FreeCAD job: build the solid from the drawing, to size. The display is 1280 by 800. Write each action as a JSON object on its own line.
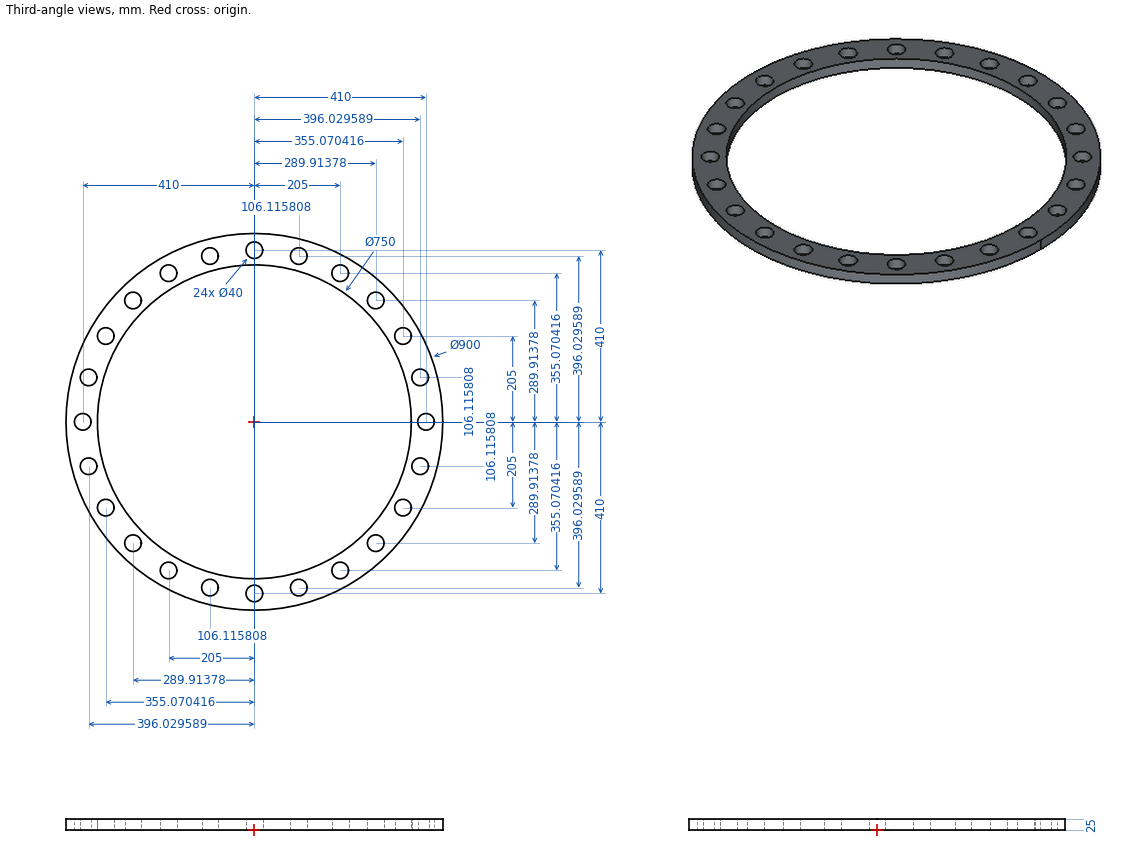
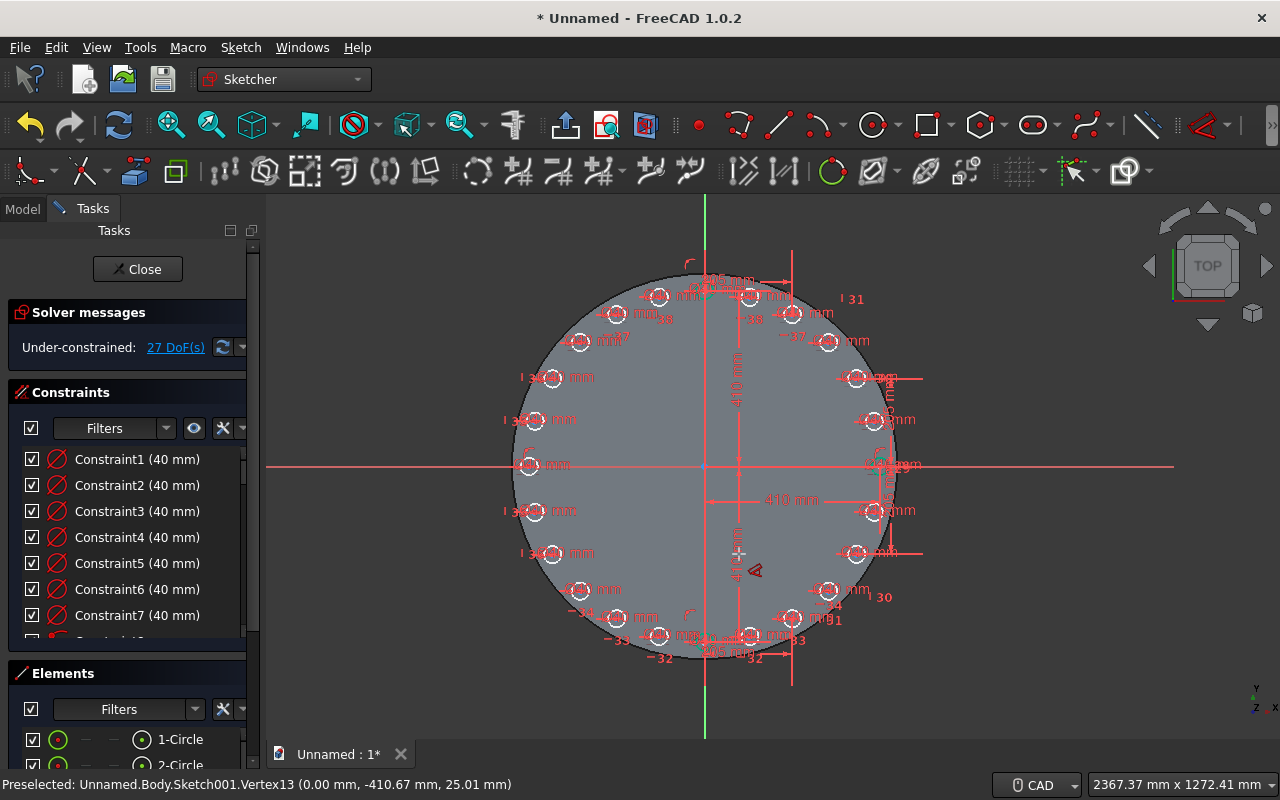
{"action": "left_click", "coordinate": [617, 619]}
{"action": "left_click", "coordinate": [640, 653]}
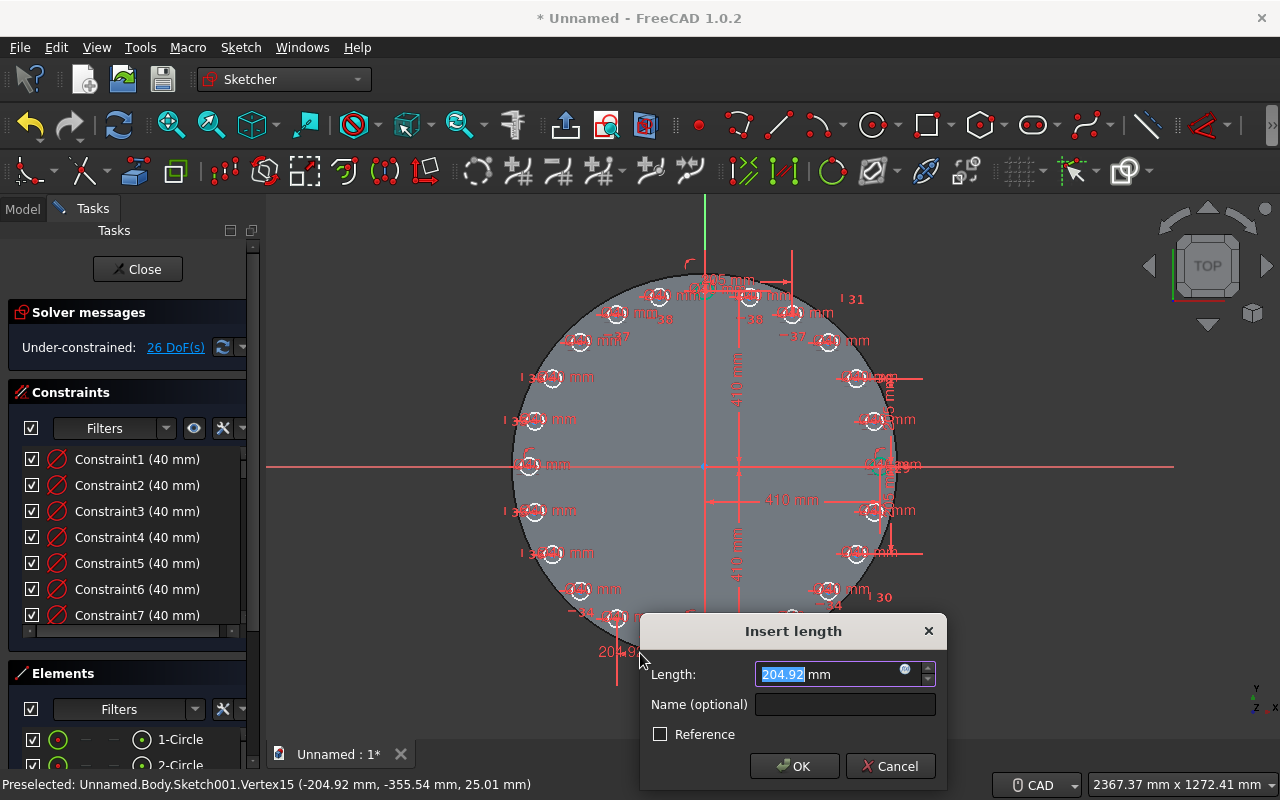
{"action": "type", "text": "205"}
{"action": "key", "text": "Return"}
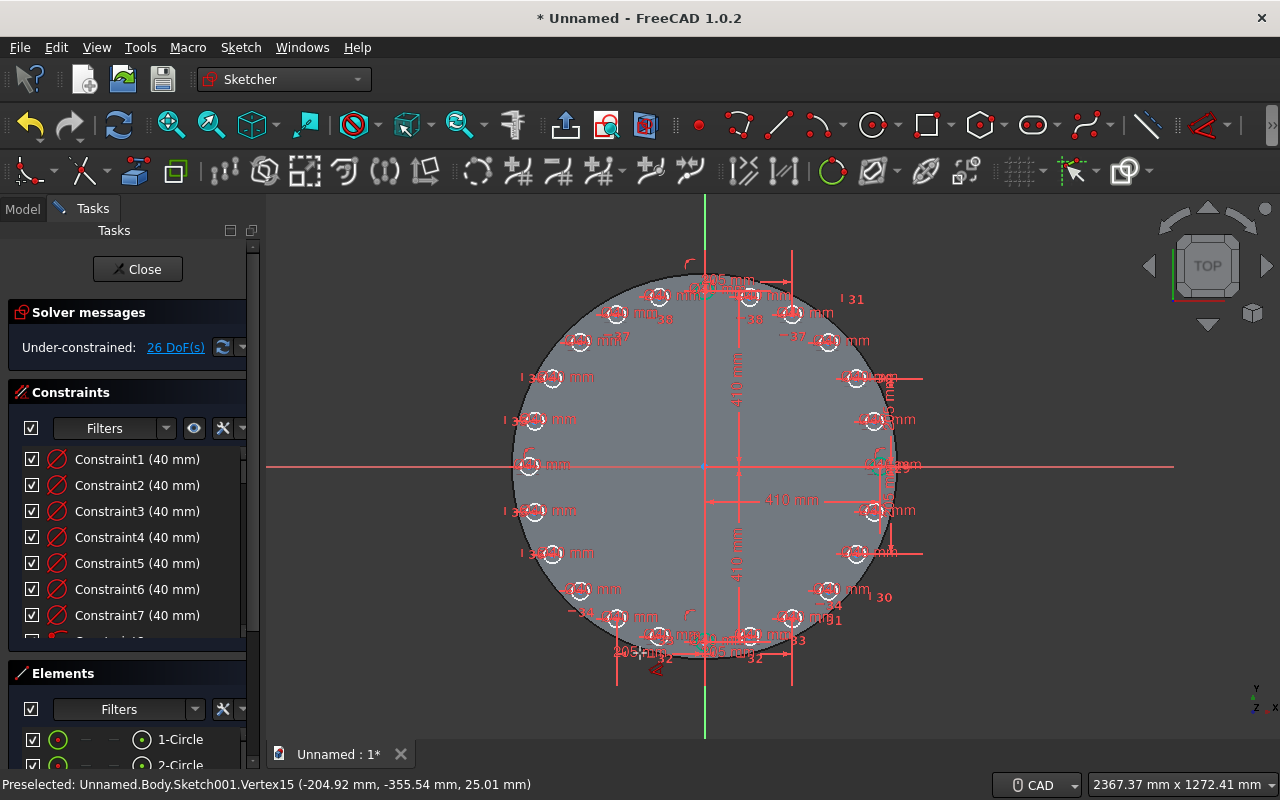
{"action": "left_click", "coordinate": [553, 555]}
{"action": "left_click", "coordinate": [519, 490]}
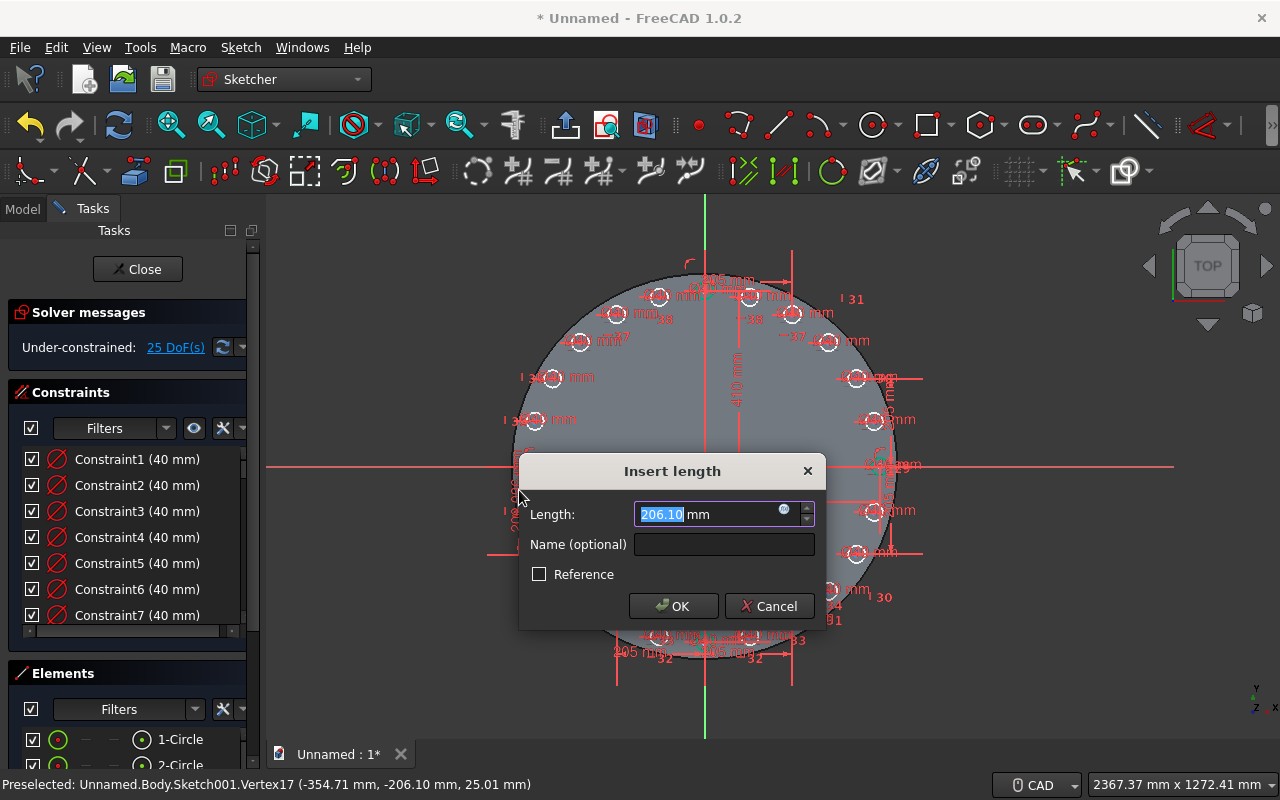
{"action": "type", "text": "205"}
{"action": "key", "text": "Return"}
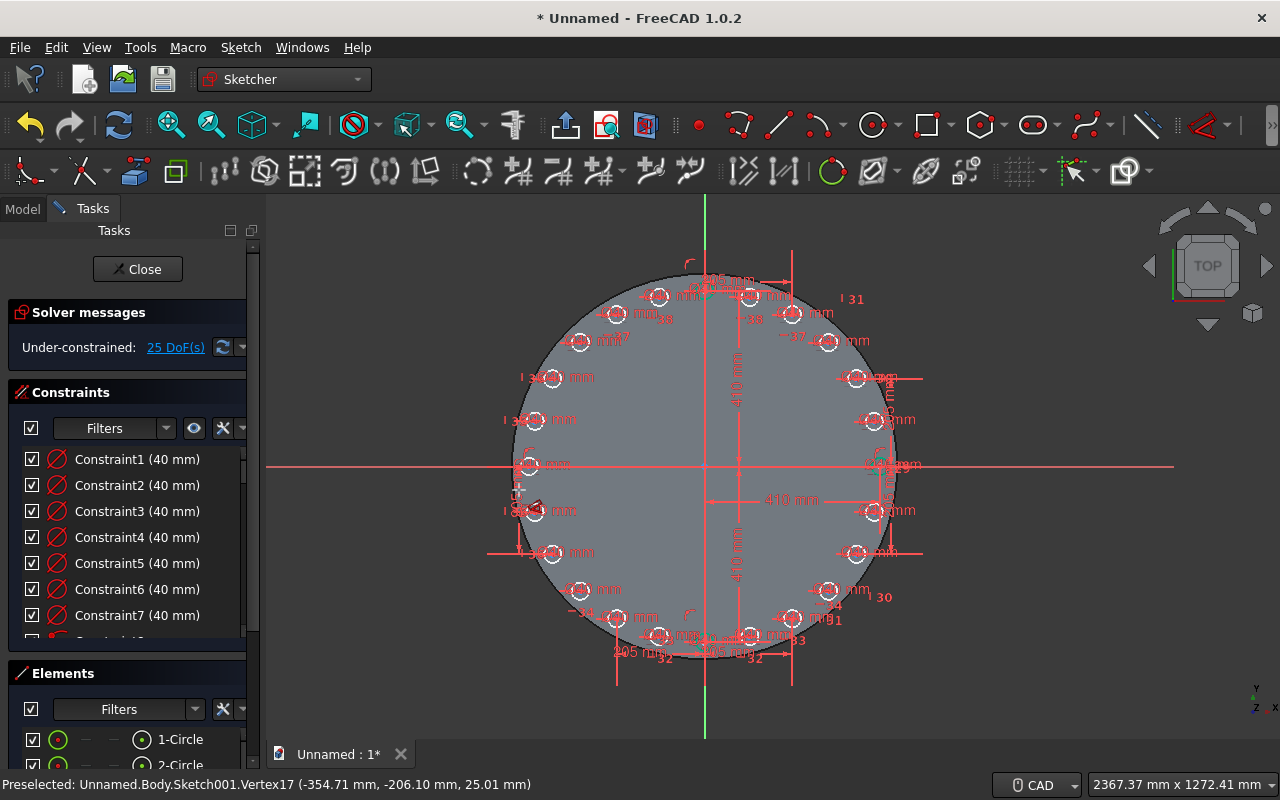
{"action": "left_click", "coordinate": [529, 467]}
{"action": "left_click", "coordinate": [617, 501]}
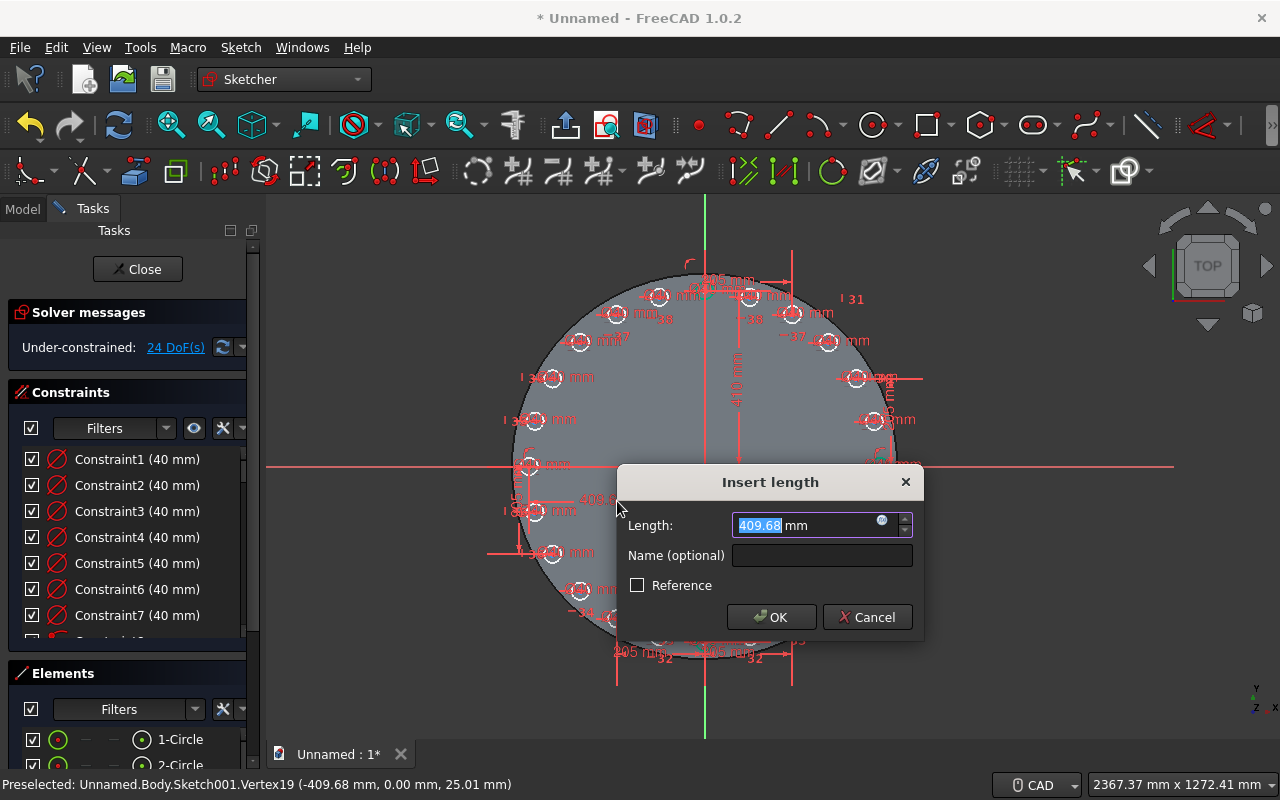
{"action": "type", "text": "410"}
{"action": "key", "text": "Return"}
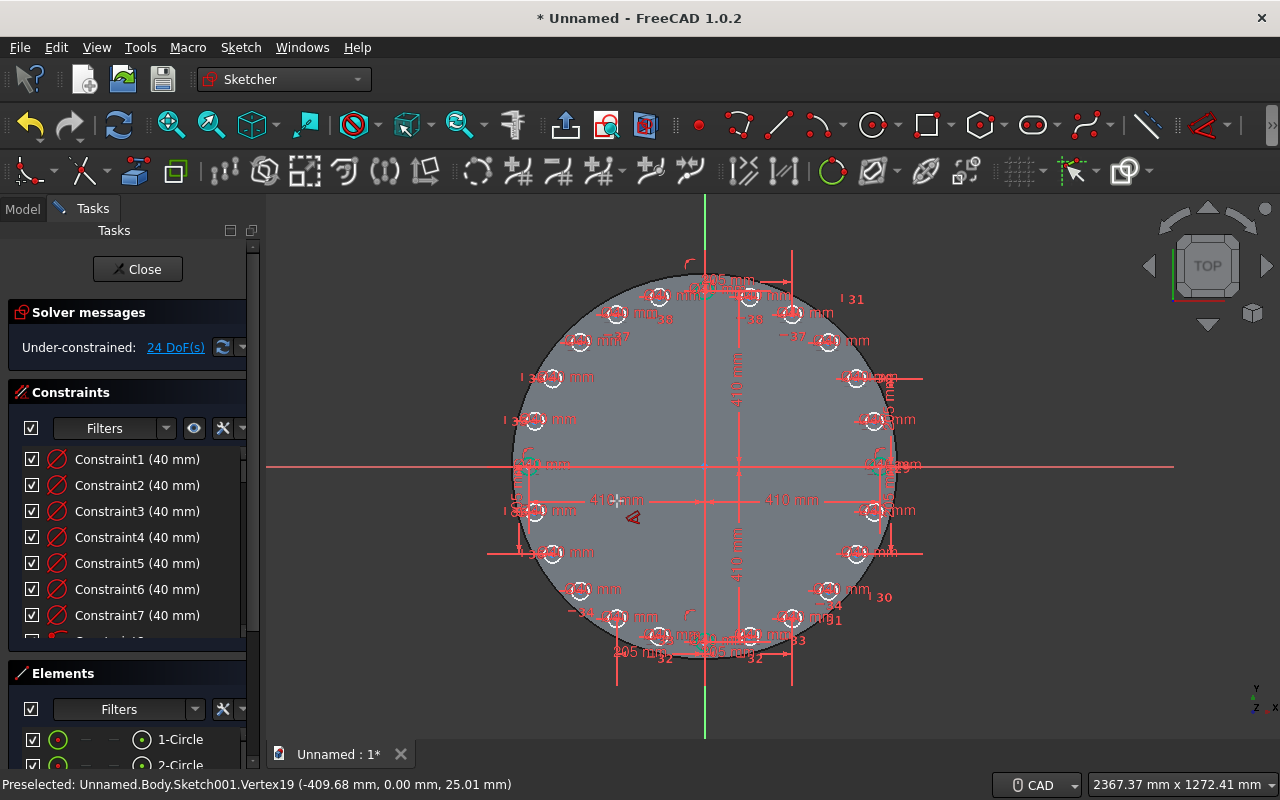
{"action": "left_click", "coordinate": [553, 379]}
{"action": "left_click", "coordinate": [519, 403]}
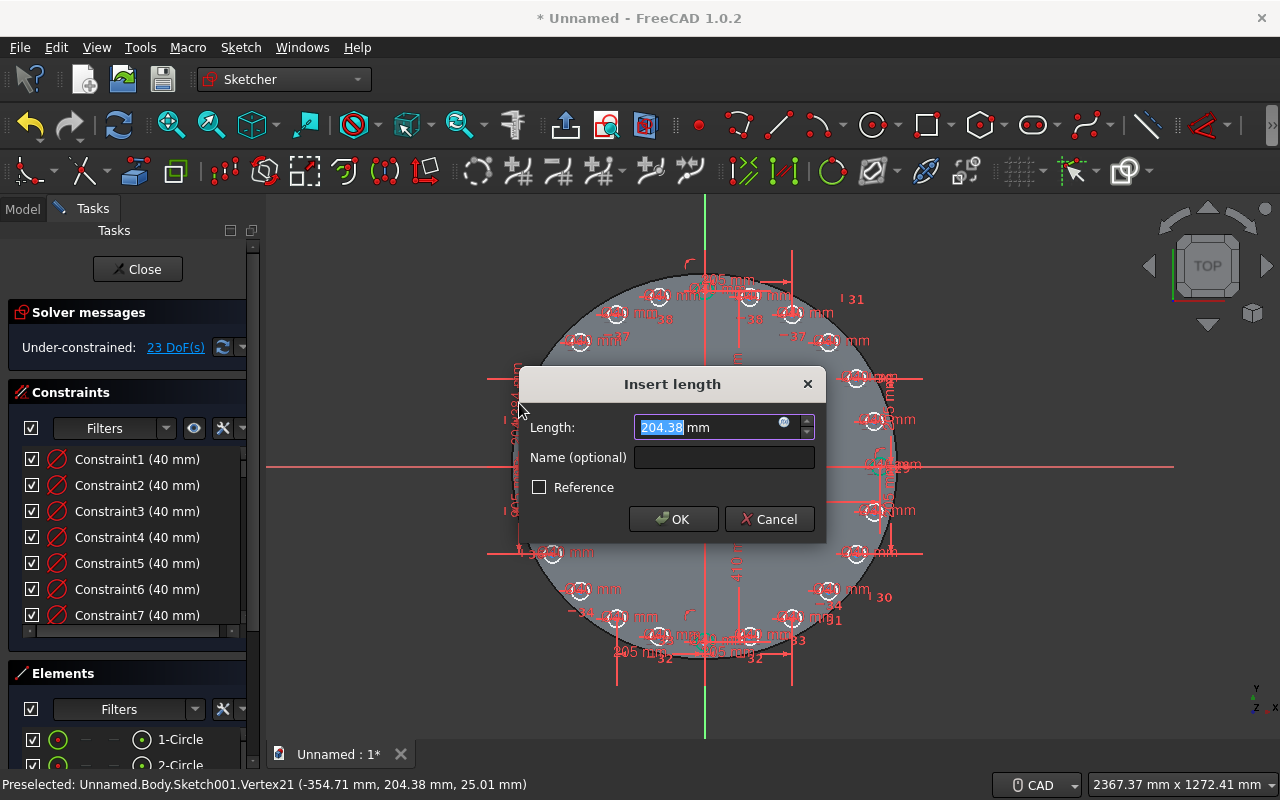
{"action": "type", "text": "205"}
{"action": "key", "text": "Return"}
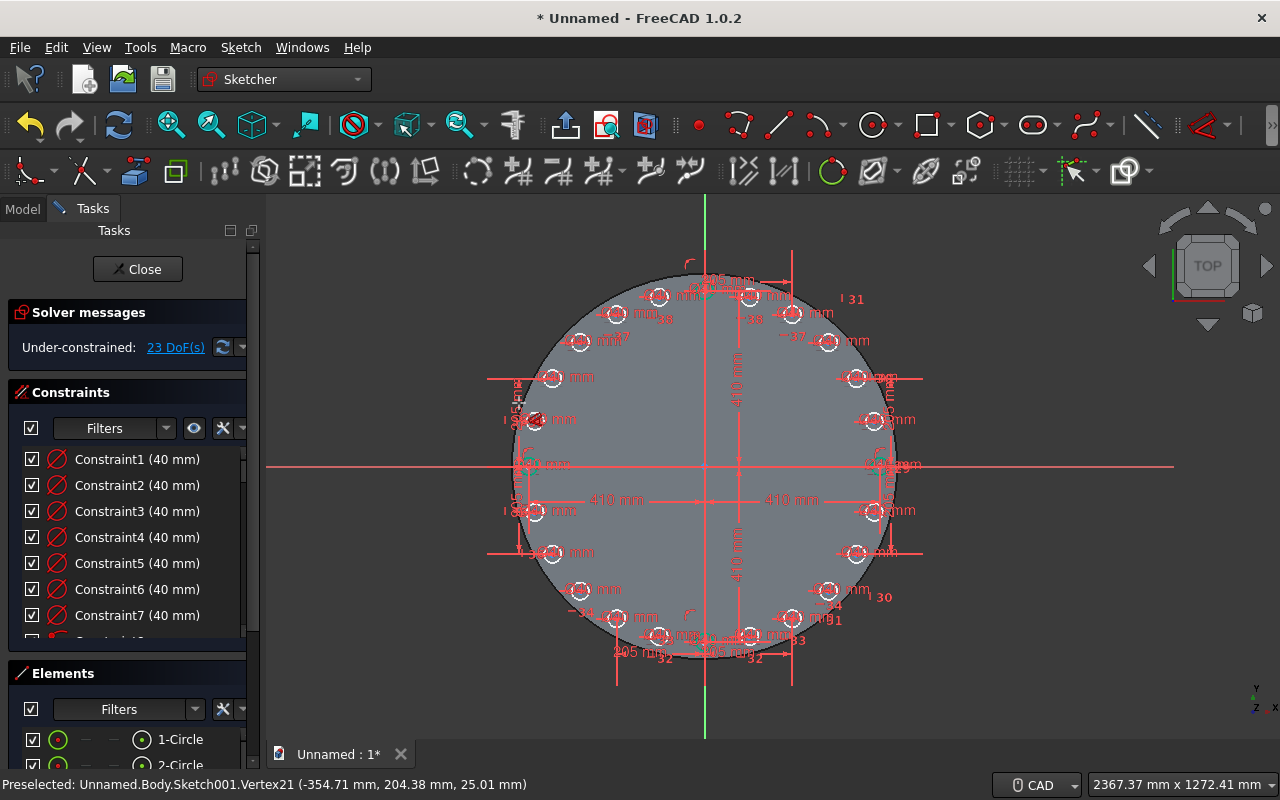
{"action": "left_click", "coordinate": [617, 315]}
{"action": "left_click", "coordinate": [640, 281]}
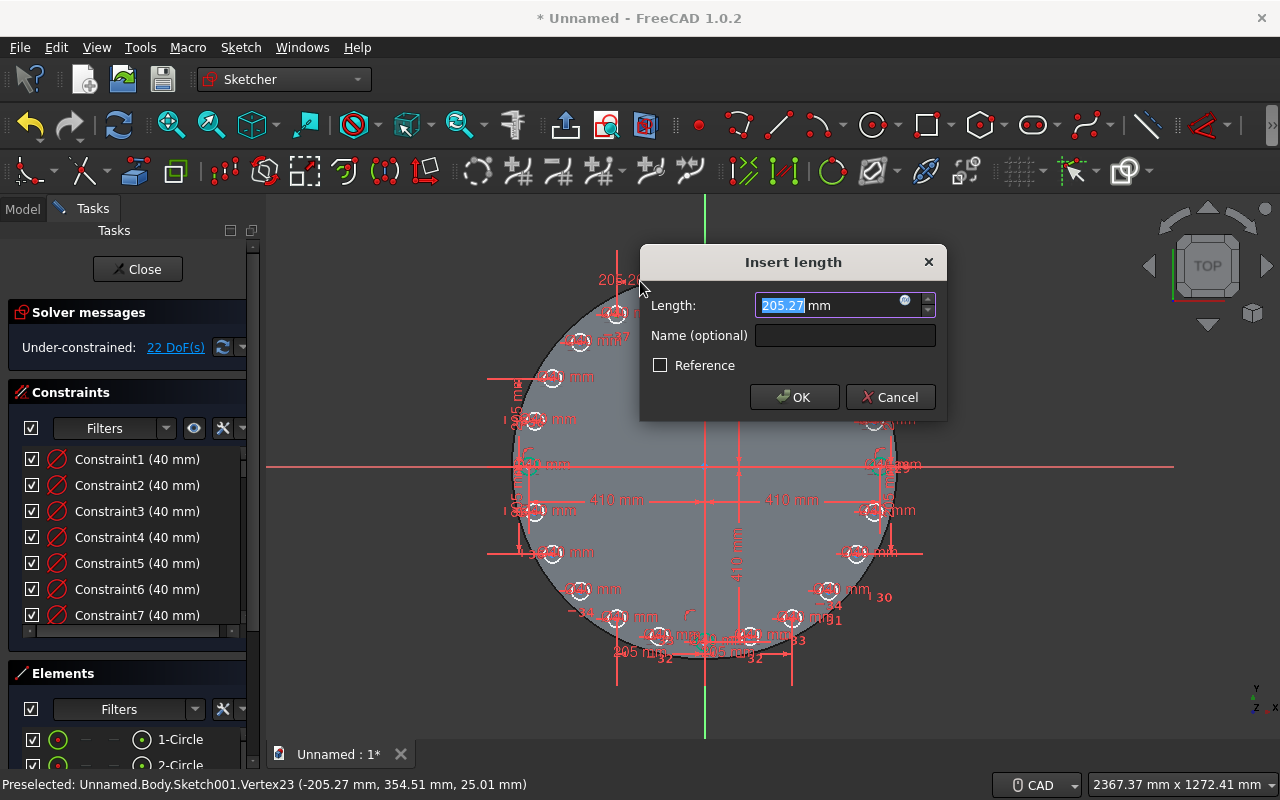
{"action": "type", "text": "205"}
{"action": "key", "text": "Return"}